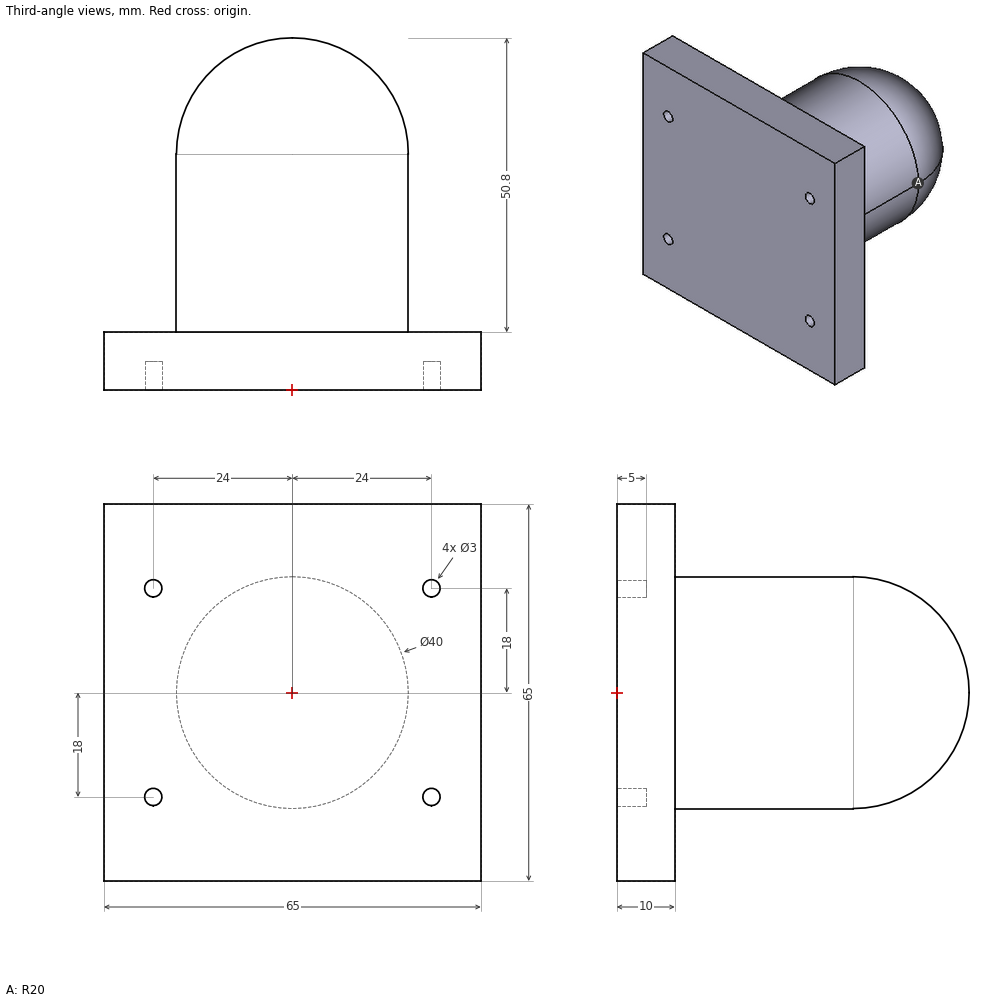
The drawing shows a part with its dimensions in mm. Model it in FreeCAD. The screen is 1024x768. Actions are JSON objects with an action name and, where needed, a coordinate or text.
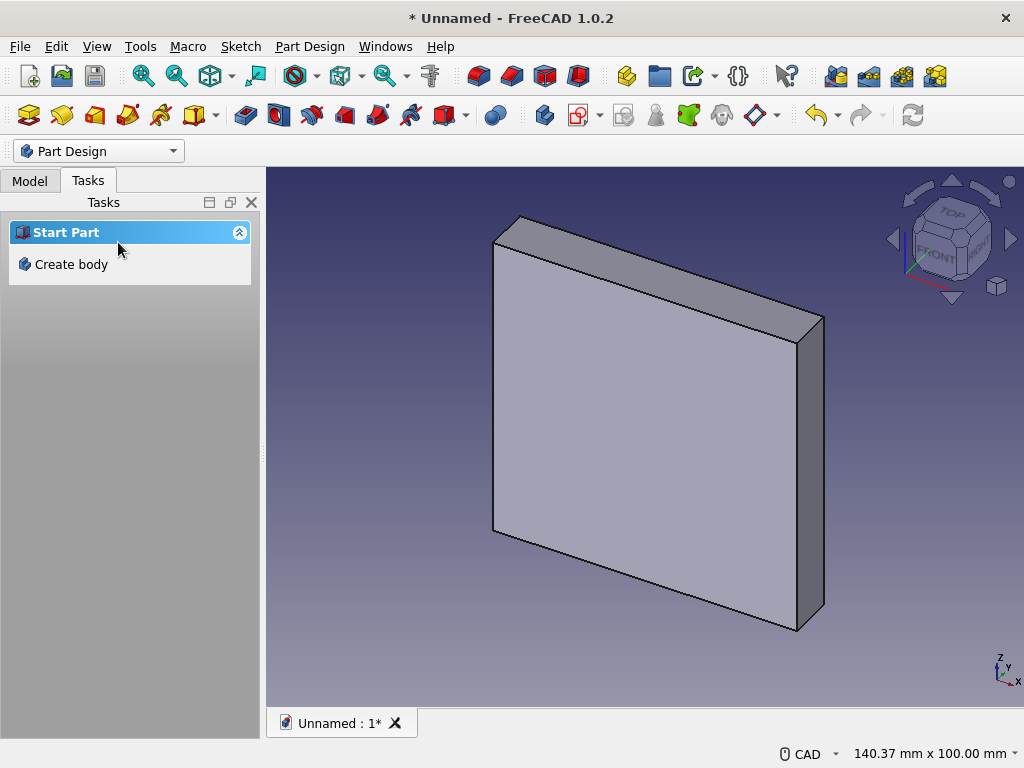
{"action": "key", "text": "4"}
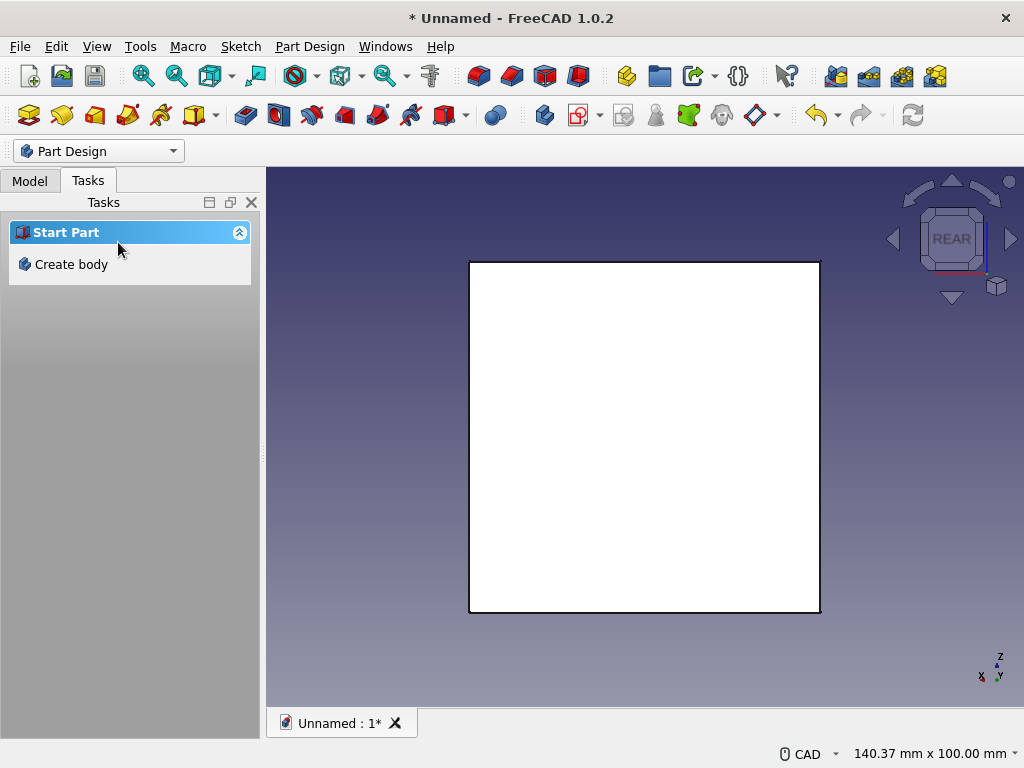
{"action": "left_click", "coordinate": [645, 436]}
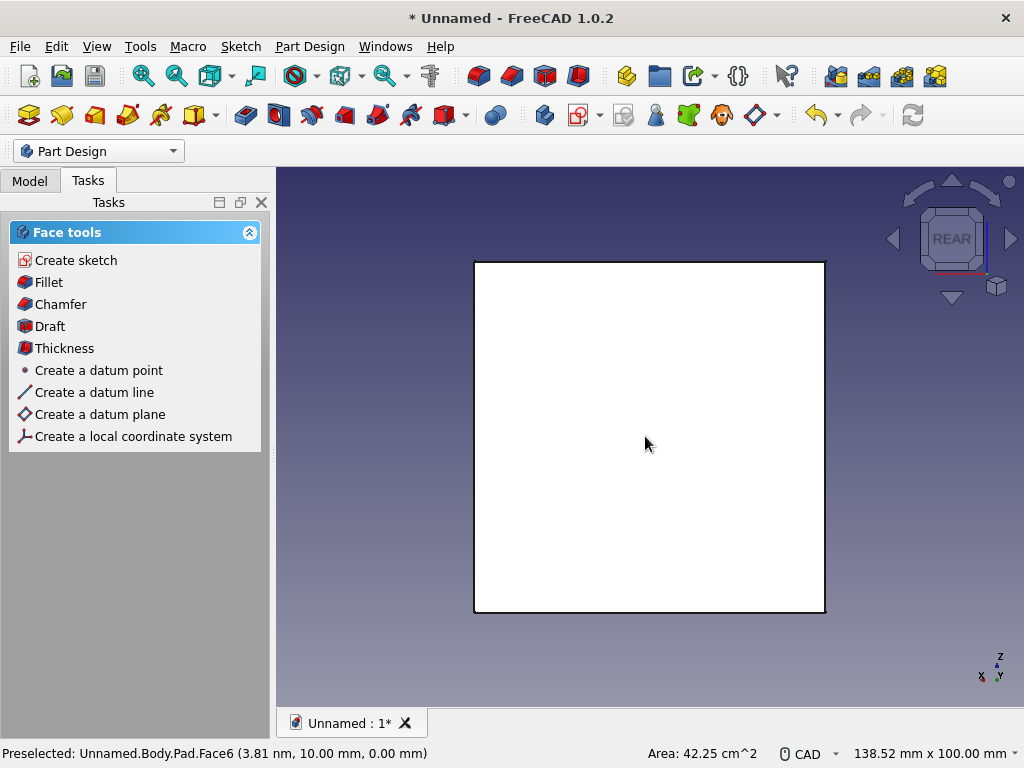
{"action": "left_click", "coordinate": [578, 116]}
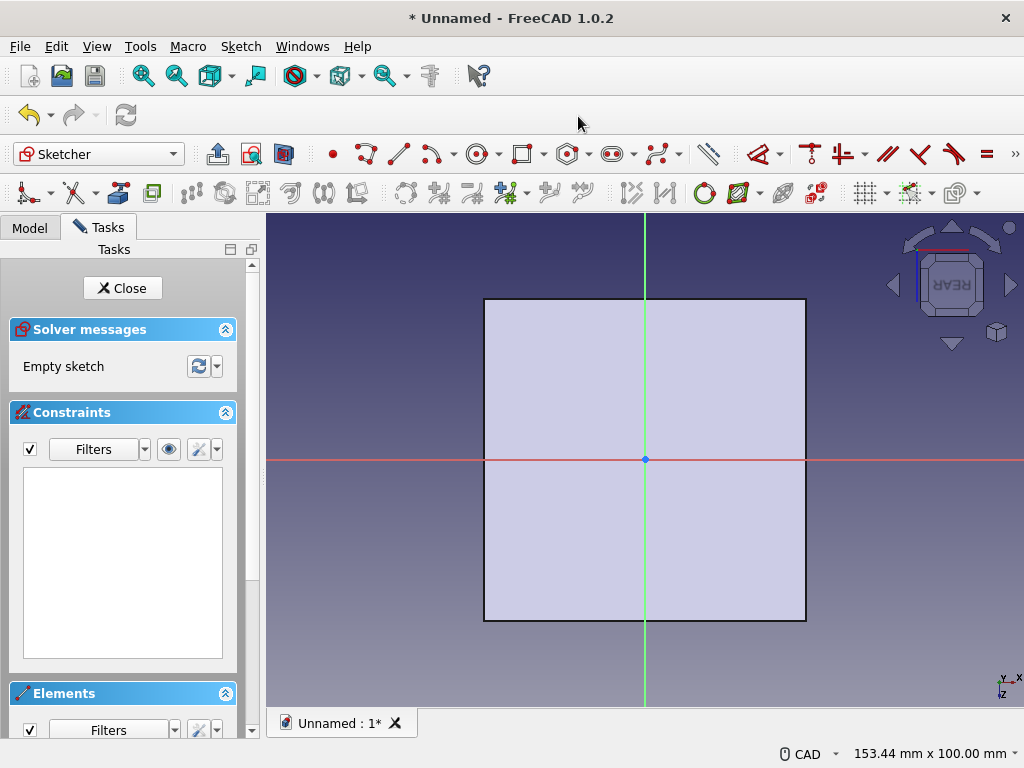
{"action": "scroll", "coordinate": [784, 460], "scroll_direction": "up", "scroll_amount": 2}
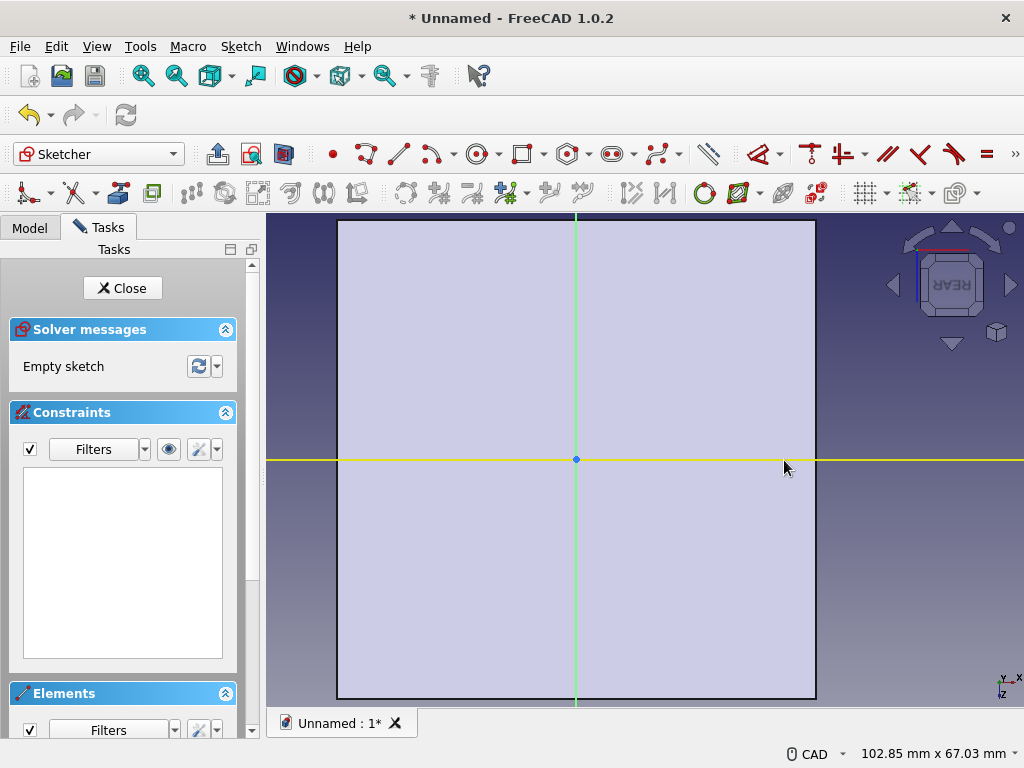
{"action": "left_click", "coordinate": [476, 154]}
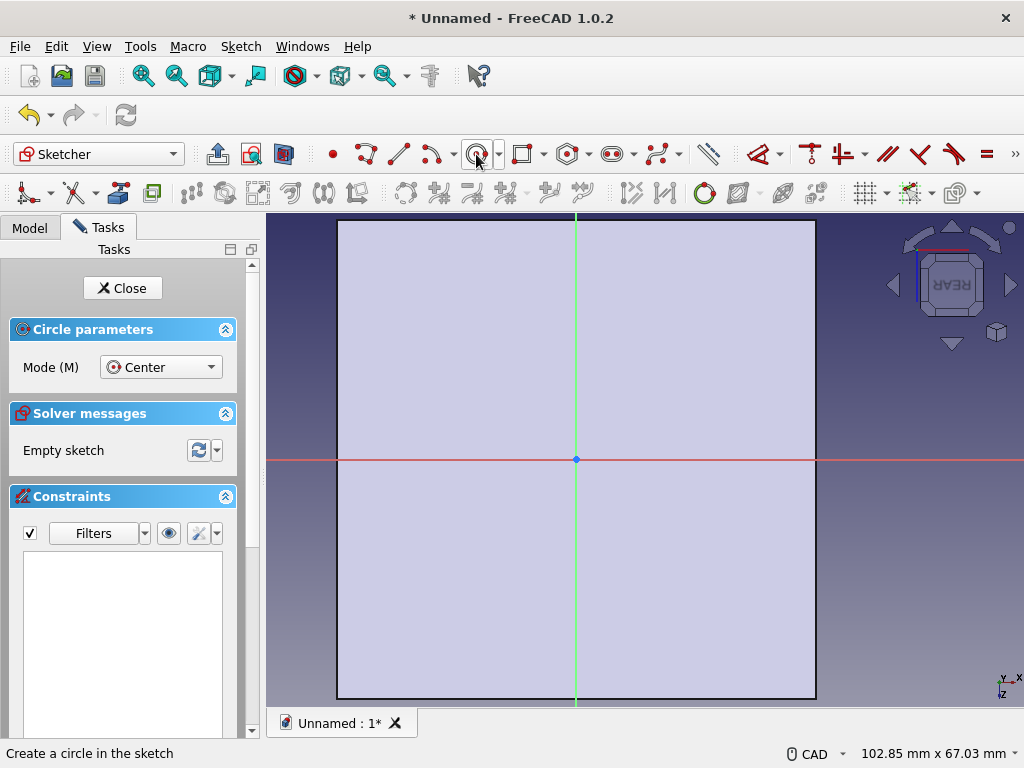
{"action": "left_click", "coordinate": [576, 460]}
{"action": "mouse_move", "coordinate": [681, 356]}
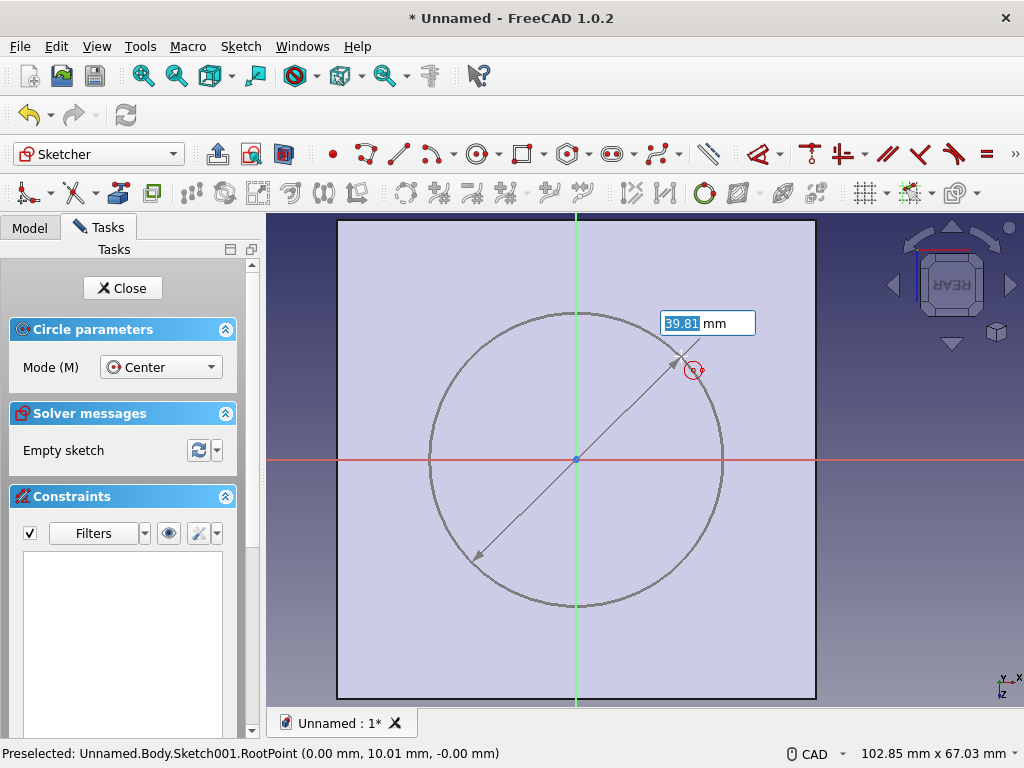
{"action": "type", "text": "40"}
{"action": "key", "text": "Return"}
{"action": "key", "text": "Escape"}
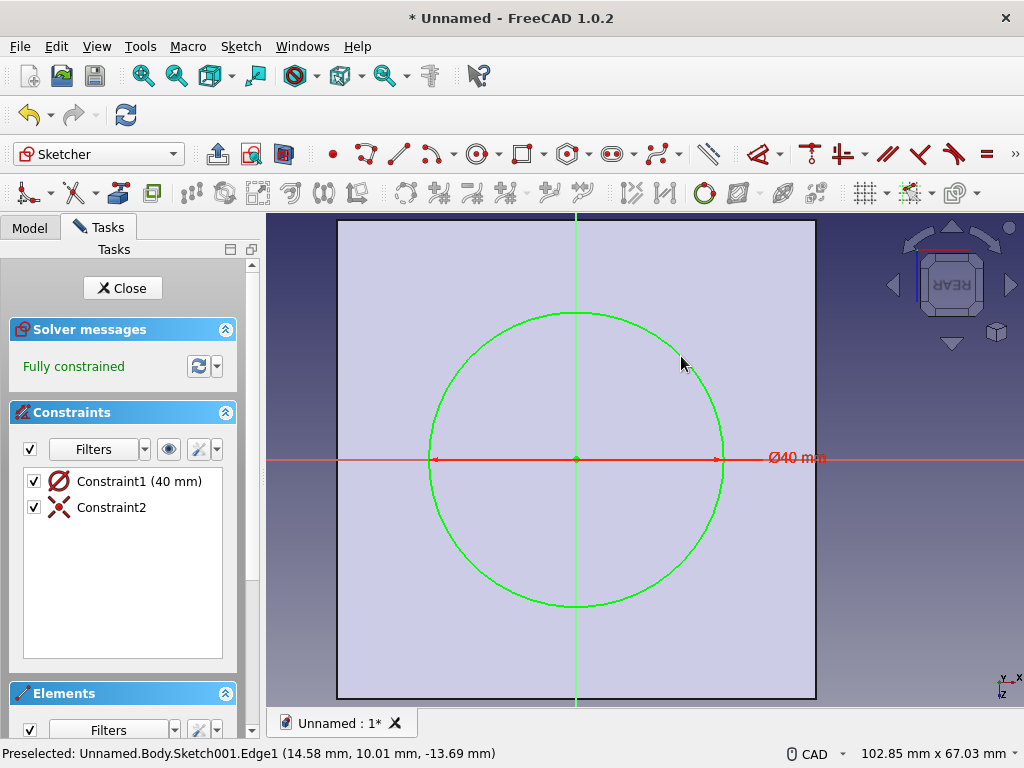
{"action": "left_click", "coordinate": [123, 288]}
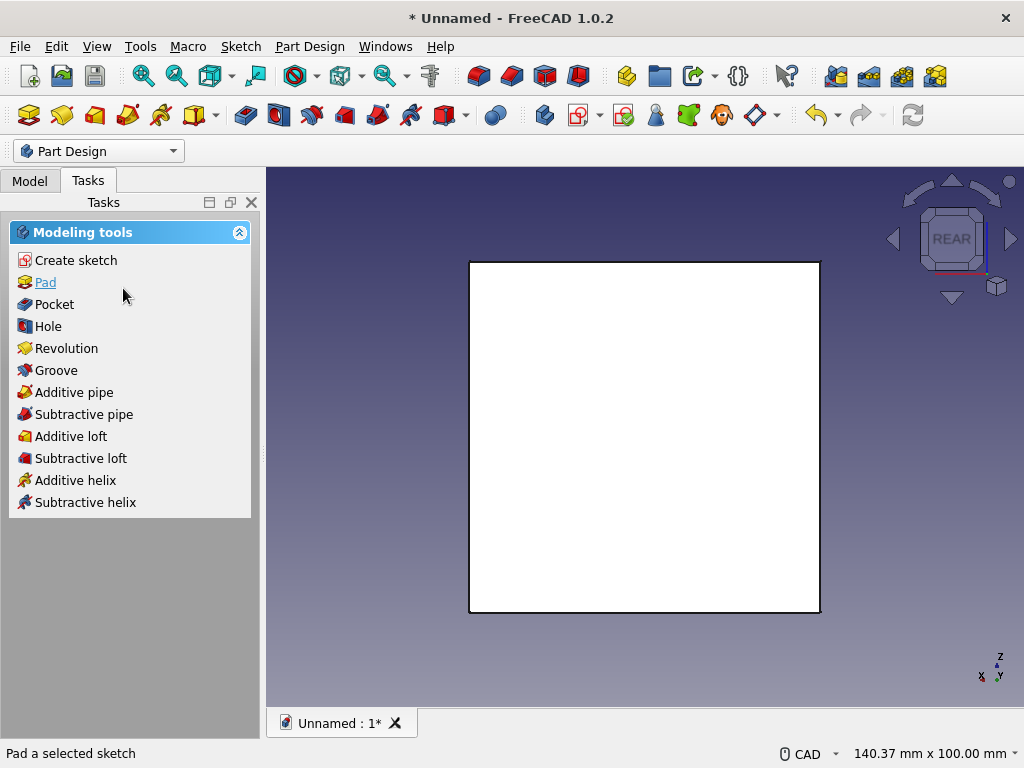
{"action": "left_click", "coordinate": [29, 116]}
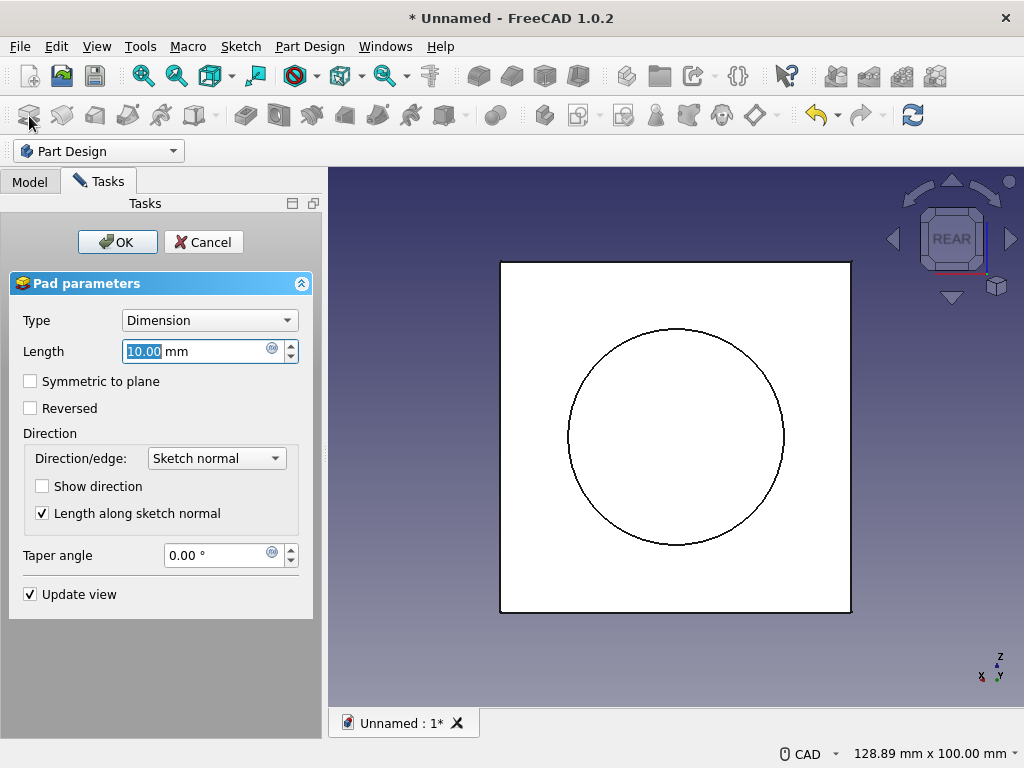
{"action": "type", "text": "50.8"}
{"action": "key", "text": "Tab"}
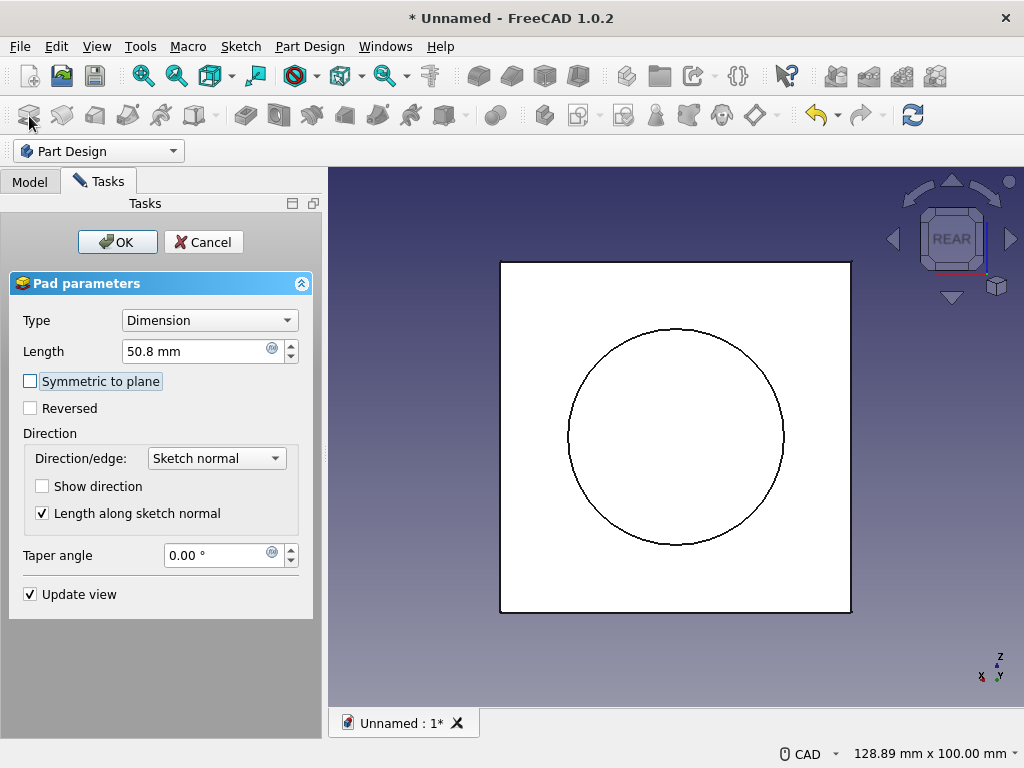
{"action": "left_click", "coordinate": [118, 242]}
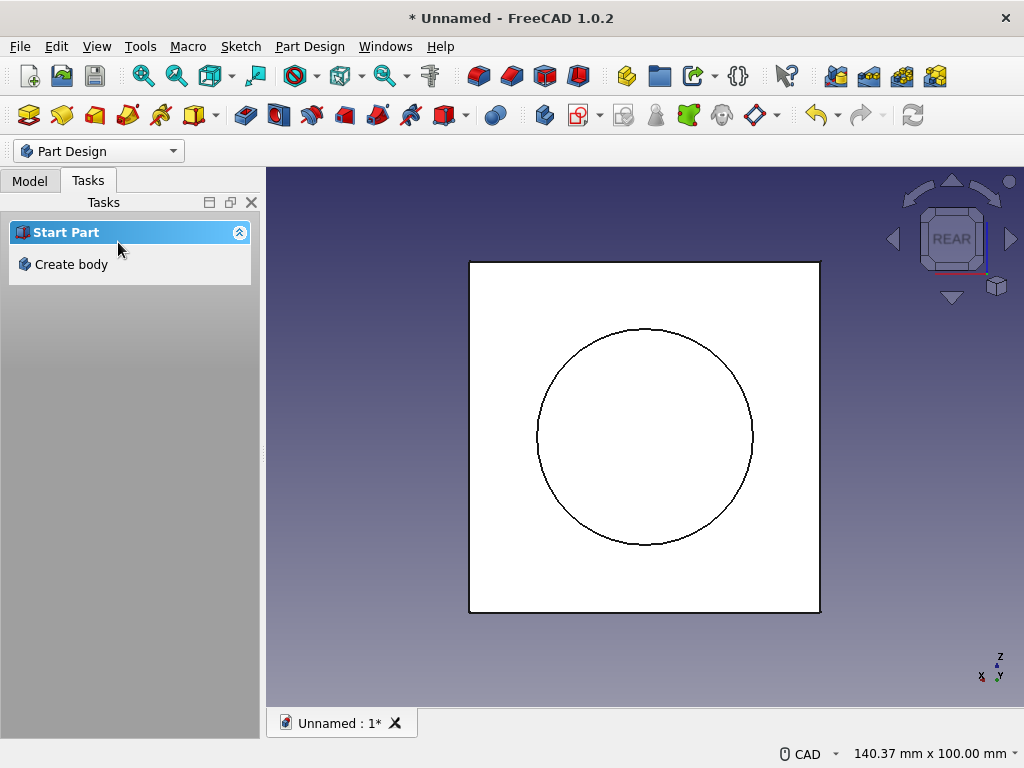
{"action": "left_click", "coordinate": [753, 436]}